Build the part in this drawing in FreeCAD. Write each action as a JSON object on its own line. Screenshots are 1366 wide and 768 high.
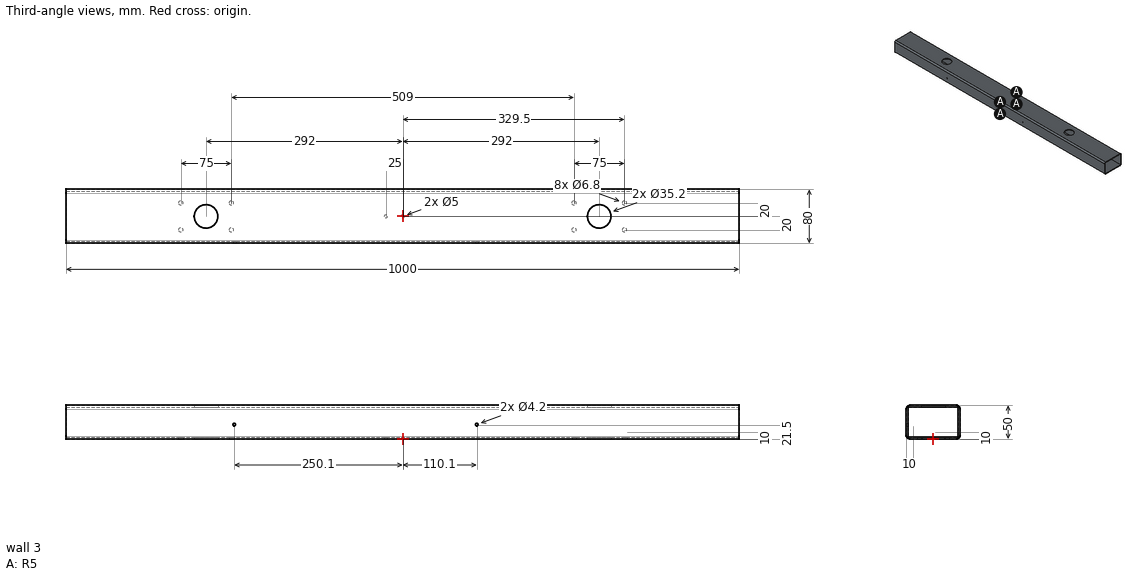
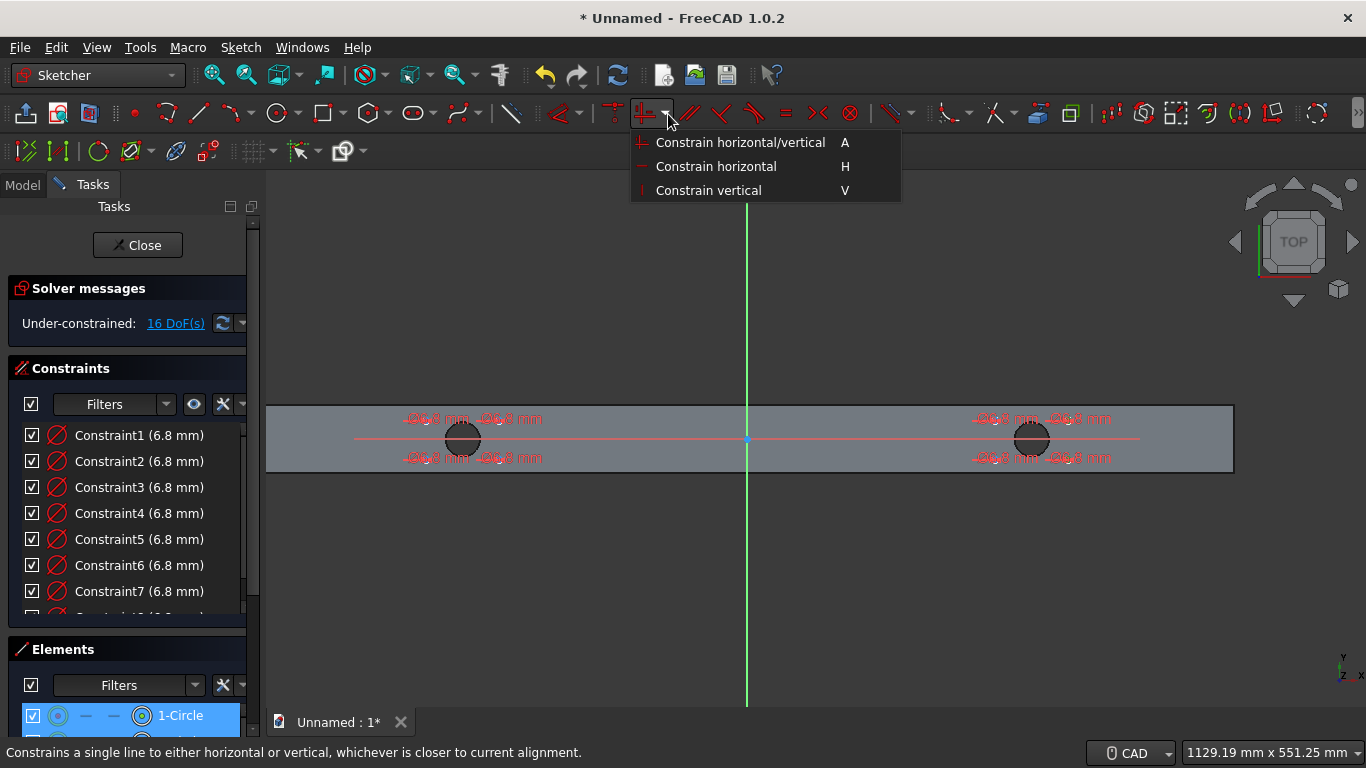
{"action": "left_click", "coordinate": [766, 190]}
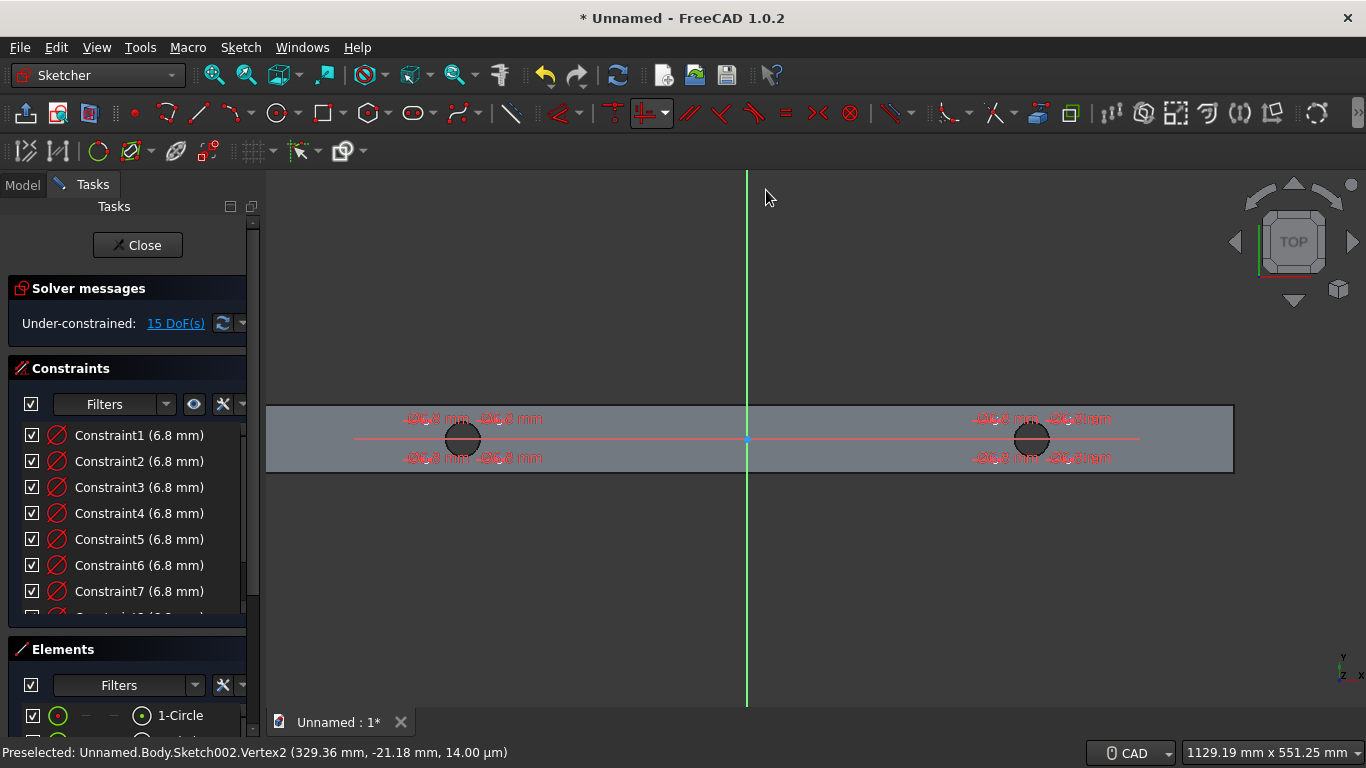
{"action": "left_click", "coordinate": [1068, 421]}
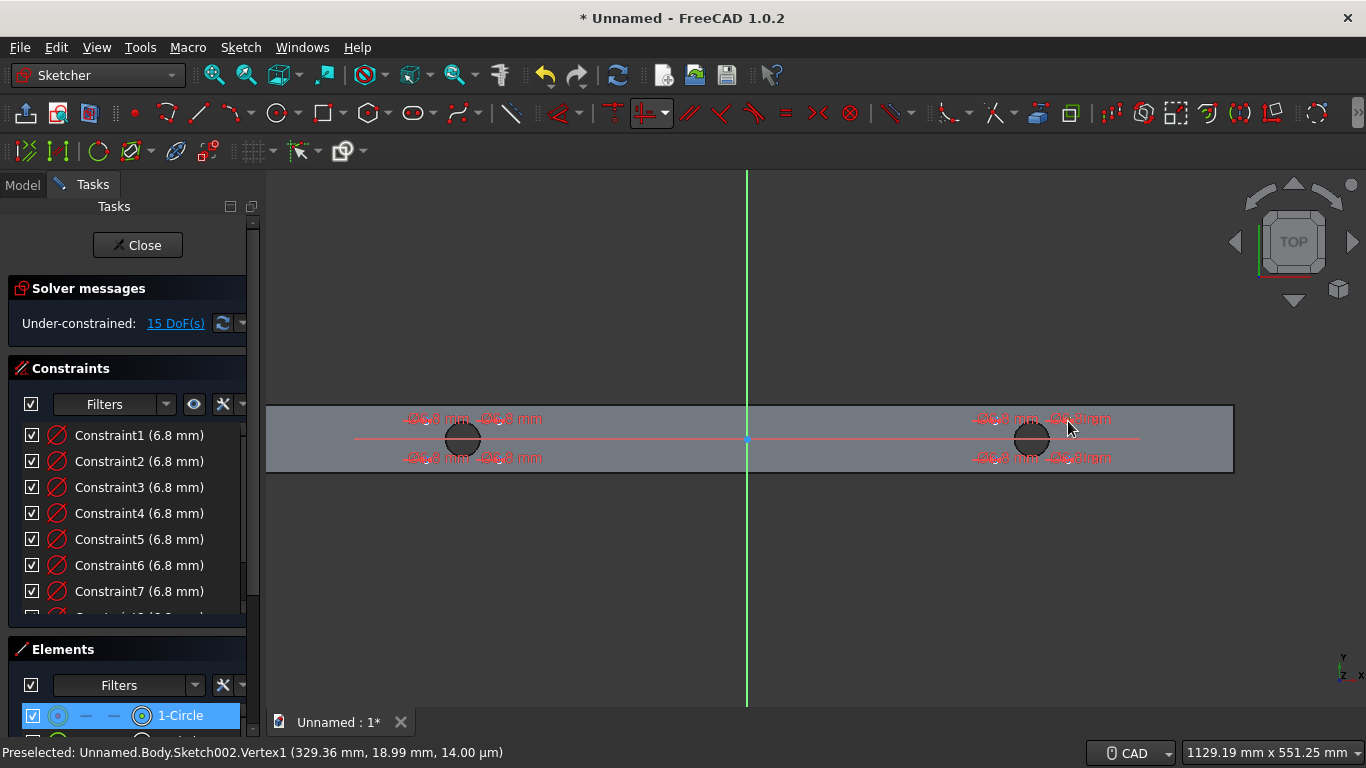
{"action": "left_click", "coordinate": [995, 421]}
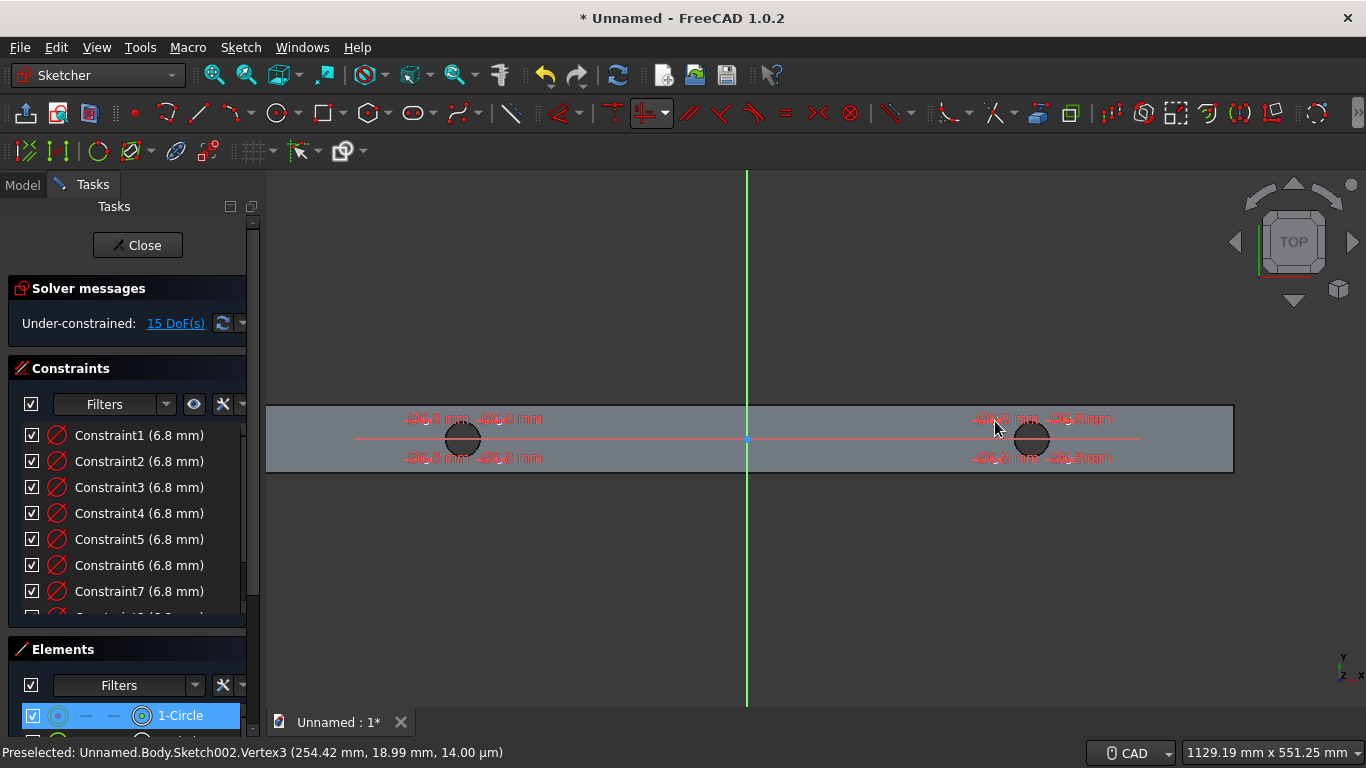
{"action": "left_click", "coordinate": [668, 114]}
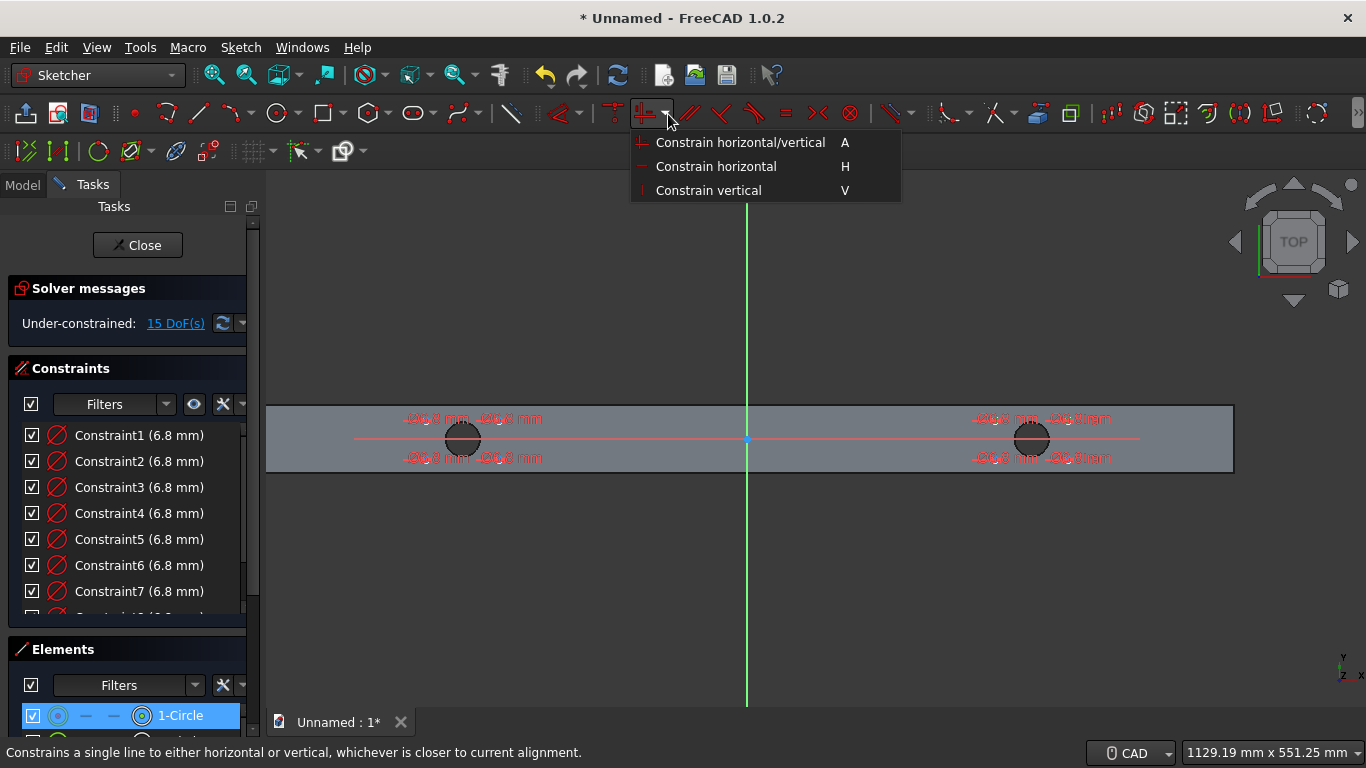
{"action": "left_click", "coordinate": [766, 166]}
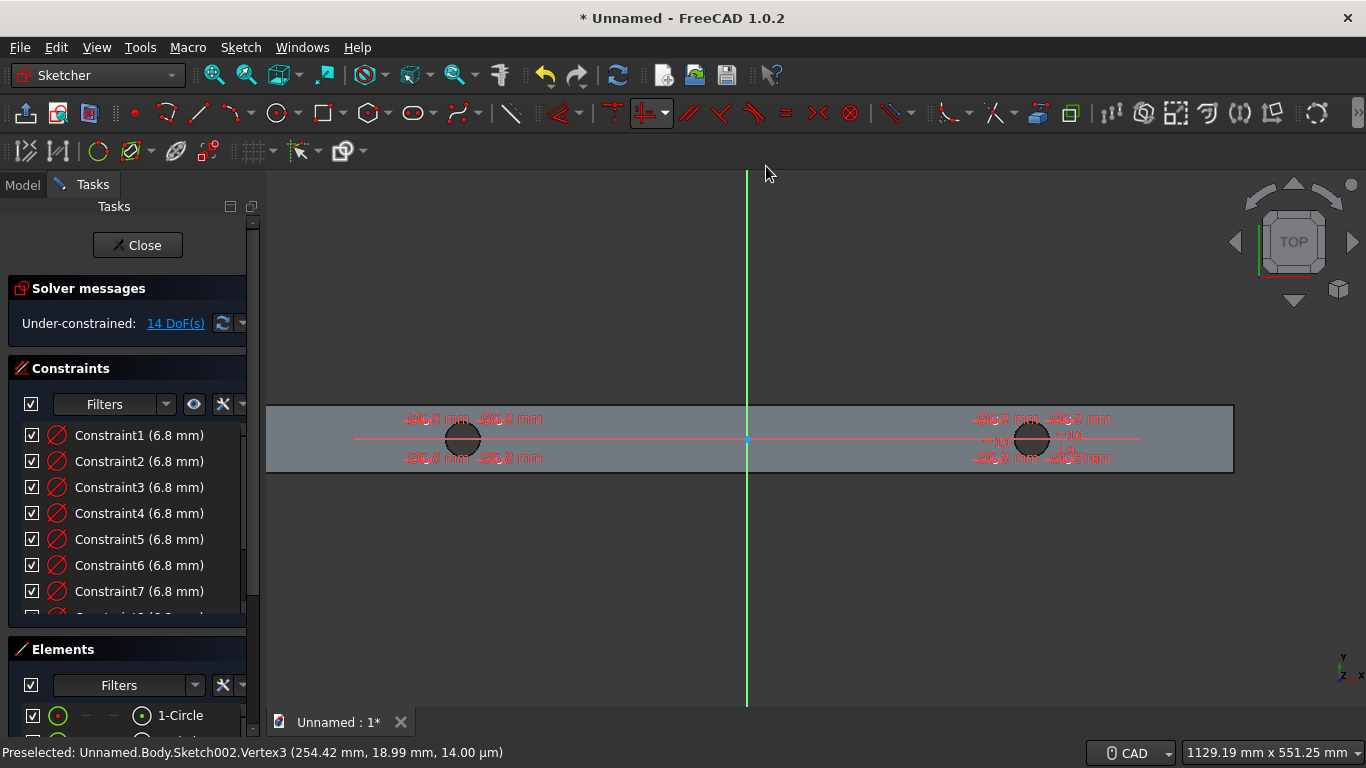
{"action": "left_click", "coordinate": [995, 421]}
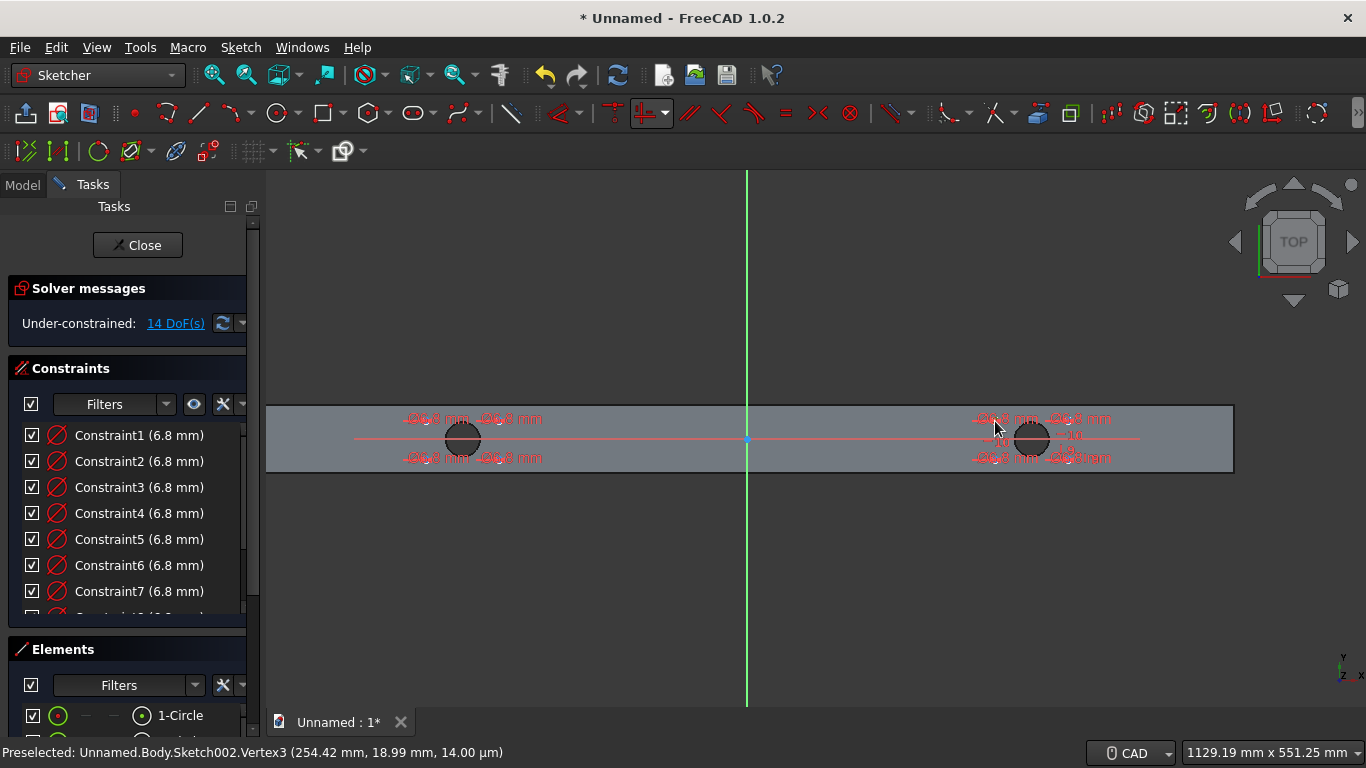
{"action": "left_click", "coordinate": [995, 460]}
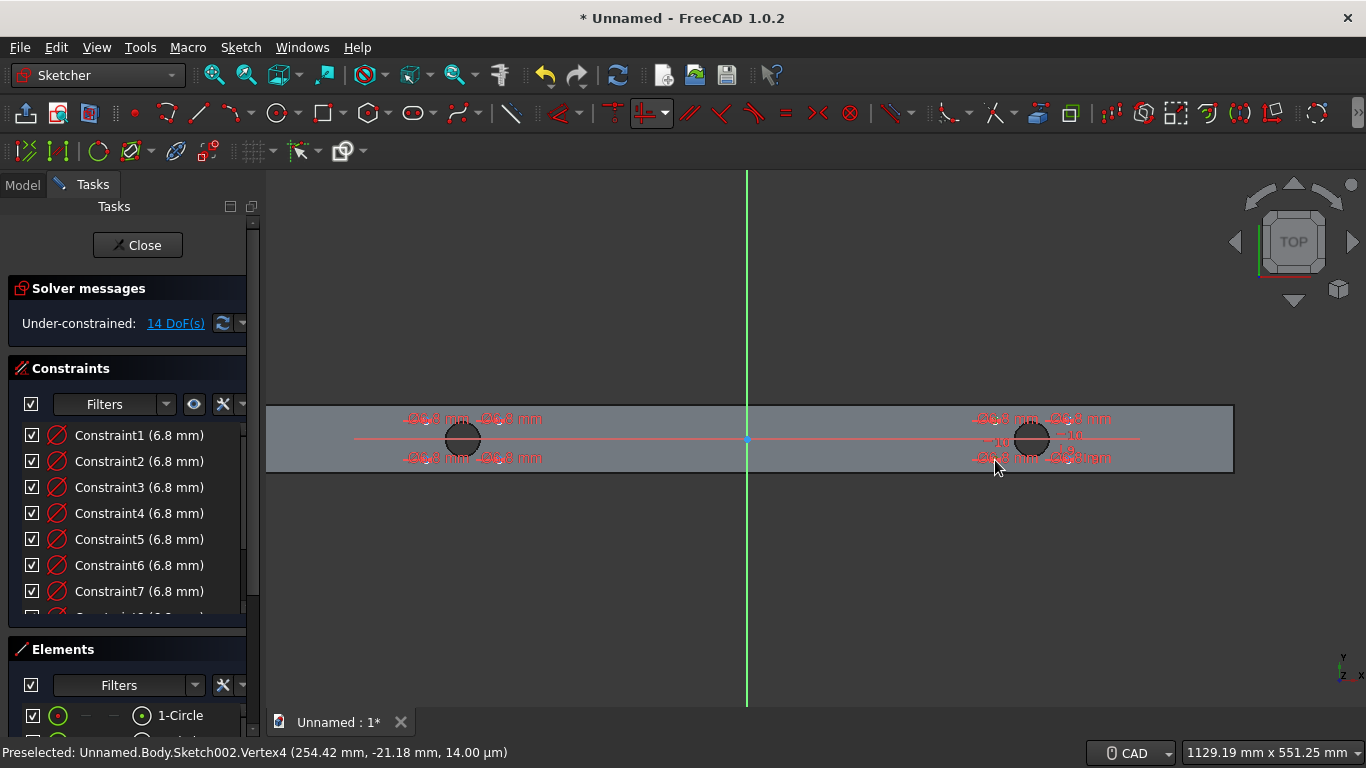
{"action": "left_click", "coordinate": [668, 114]}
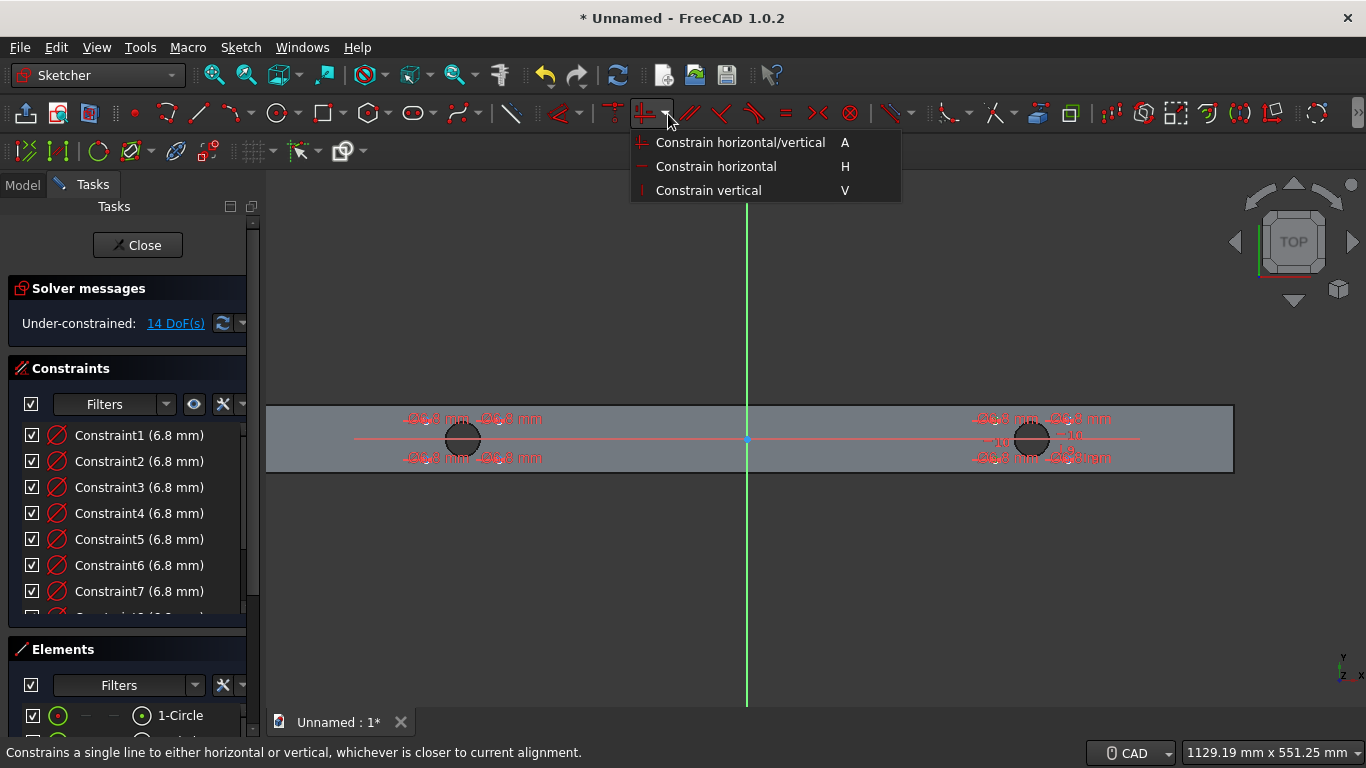
{"action": "left_click", "coordinate": [766, 190]}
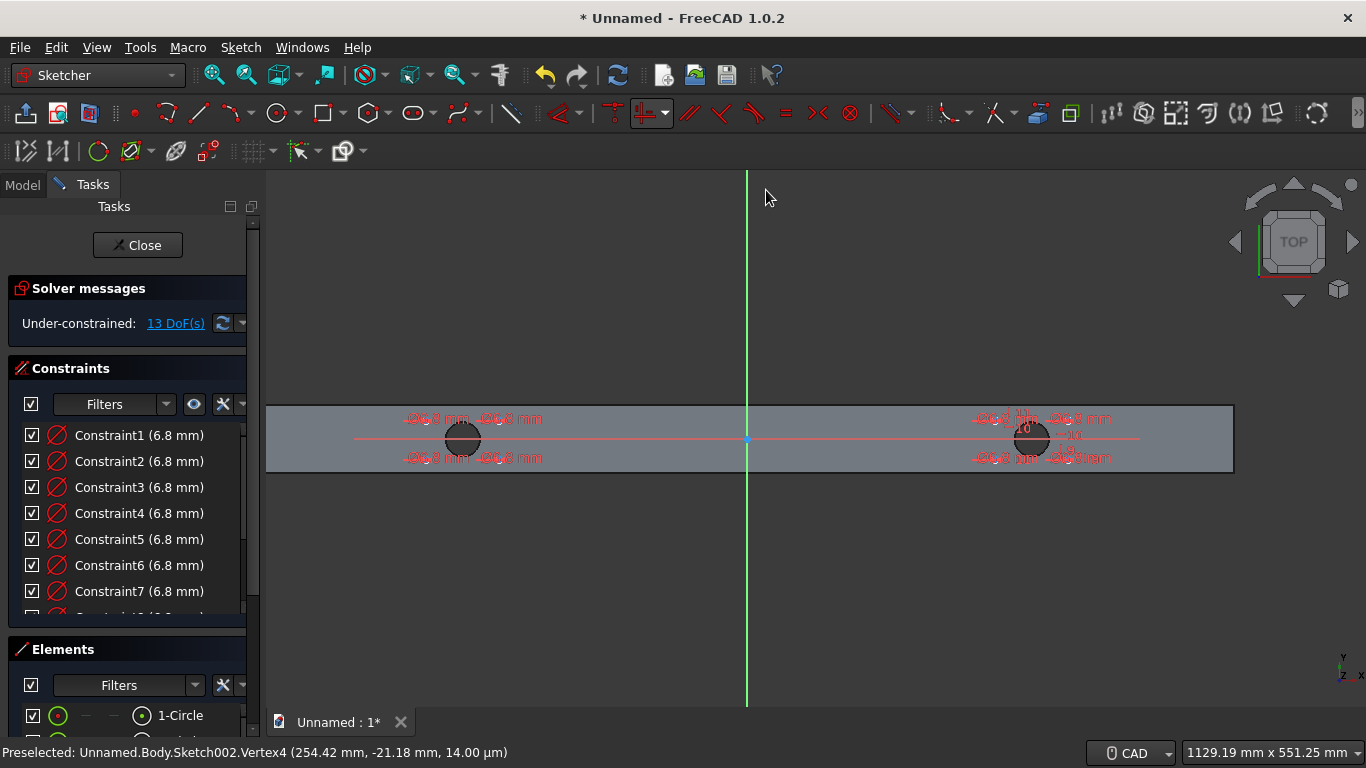
{"action": "left_click", "coordinate": [1068, 460]}